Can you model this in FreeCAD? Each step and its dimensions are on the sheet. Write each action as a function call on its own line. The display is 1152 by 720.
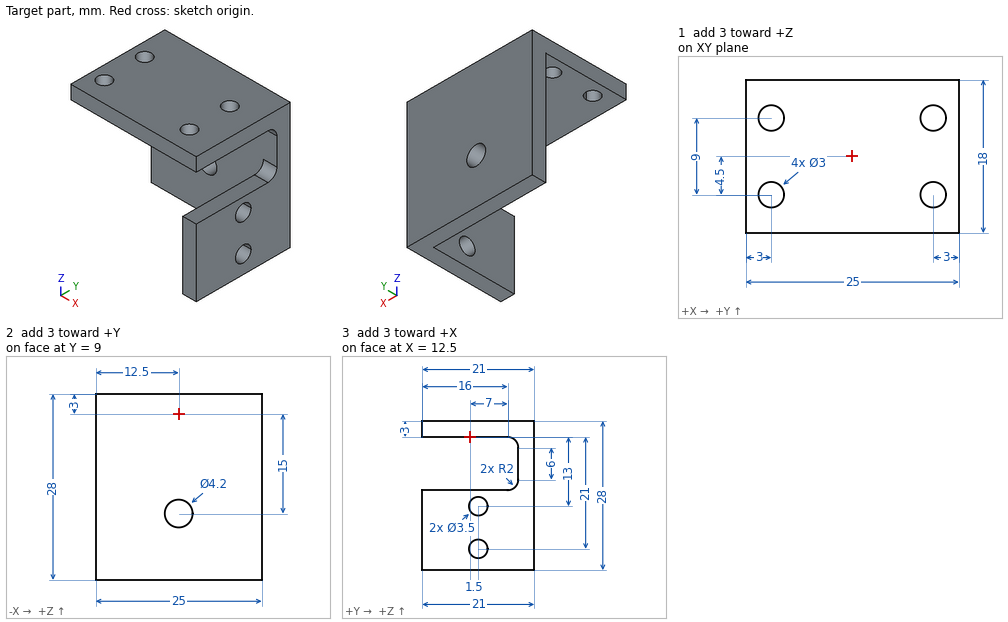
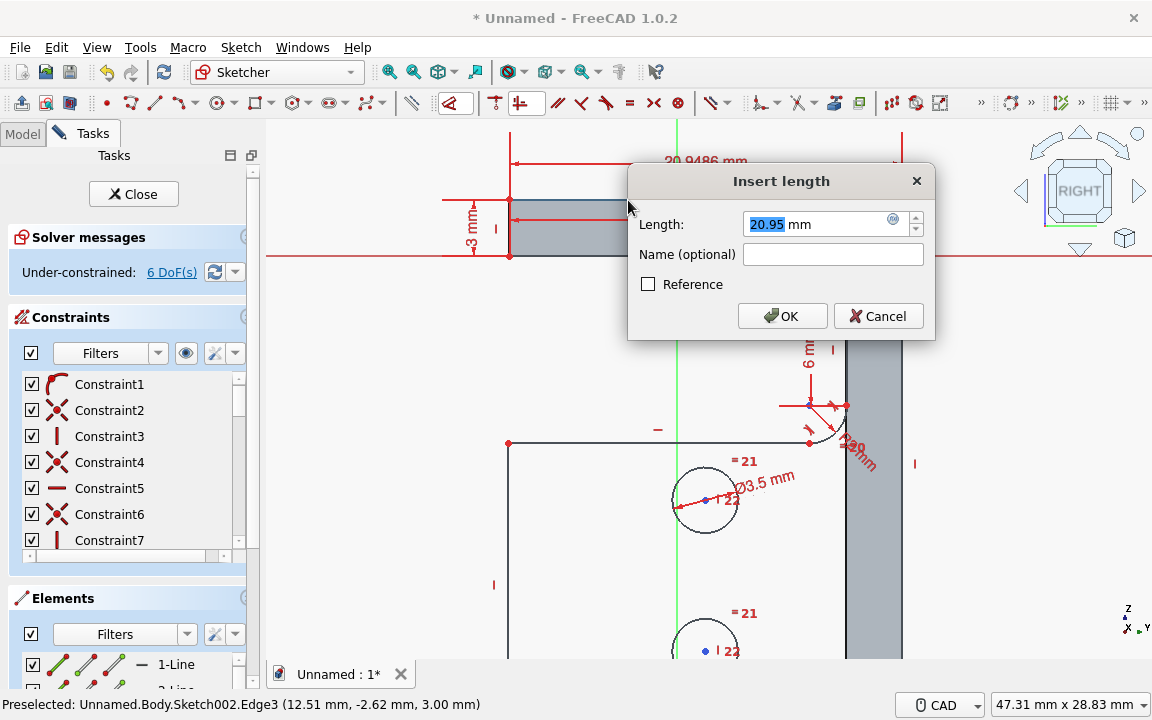
text(21)
key(Return)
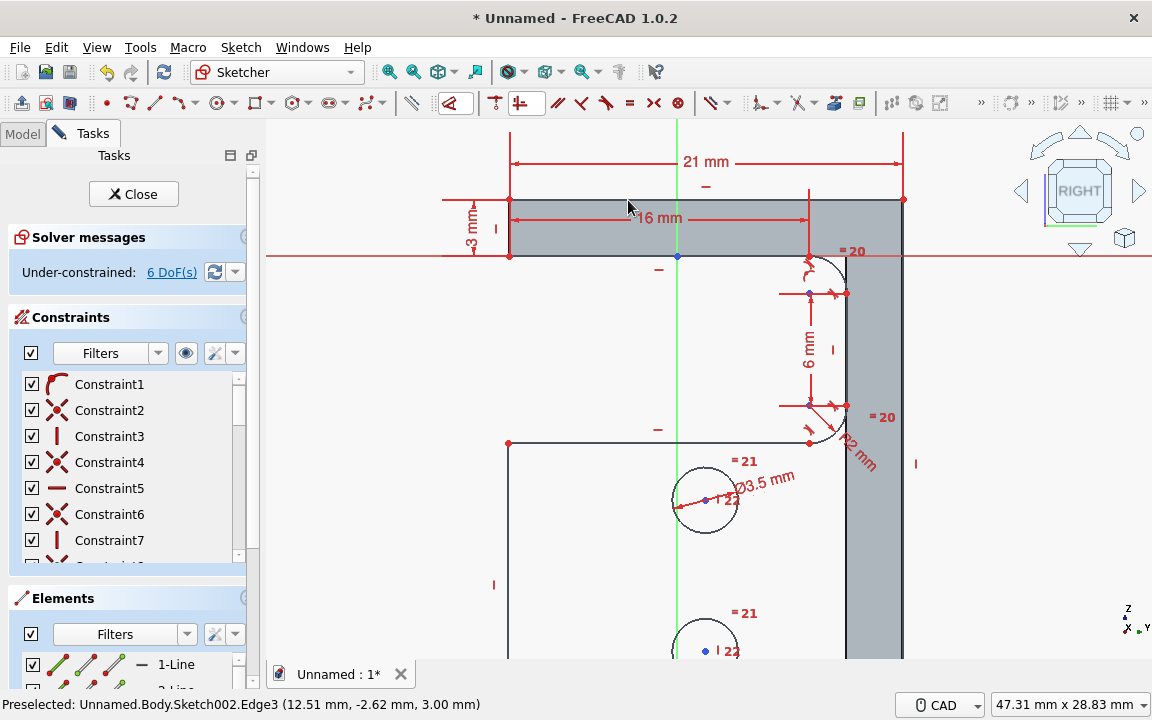
click(903, 358)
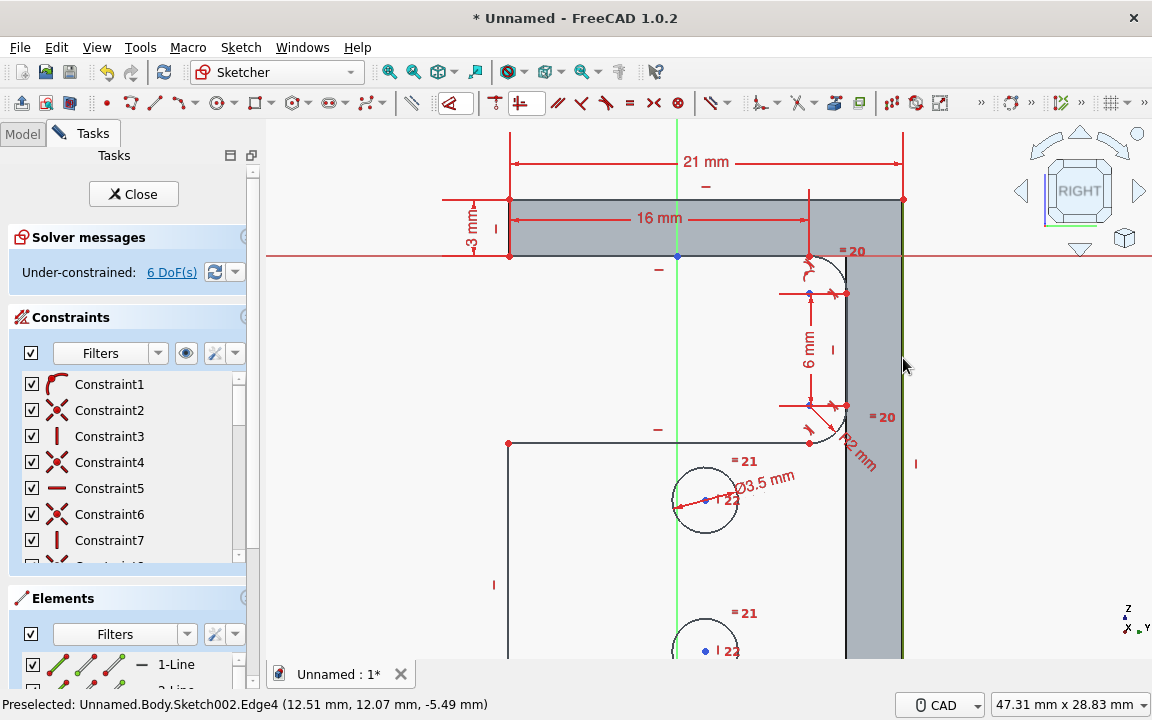
key(i)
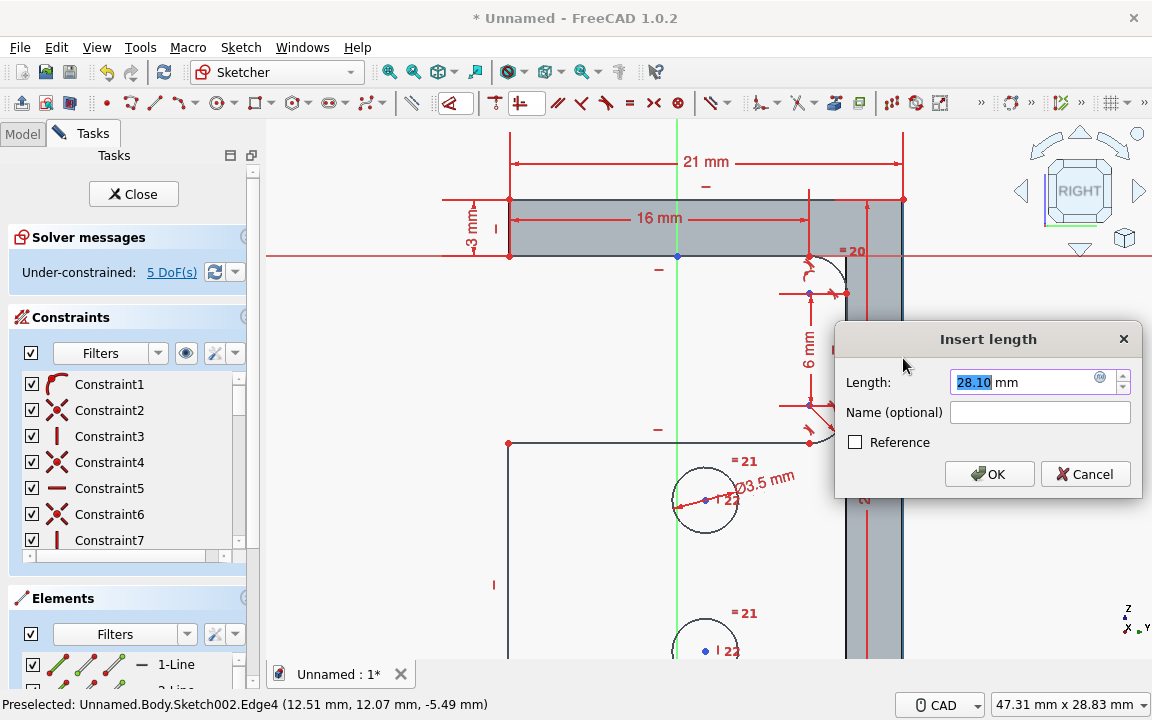
text(28)
key(Return)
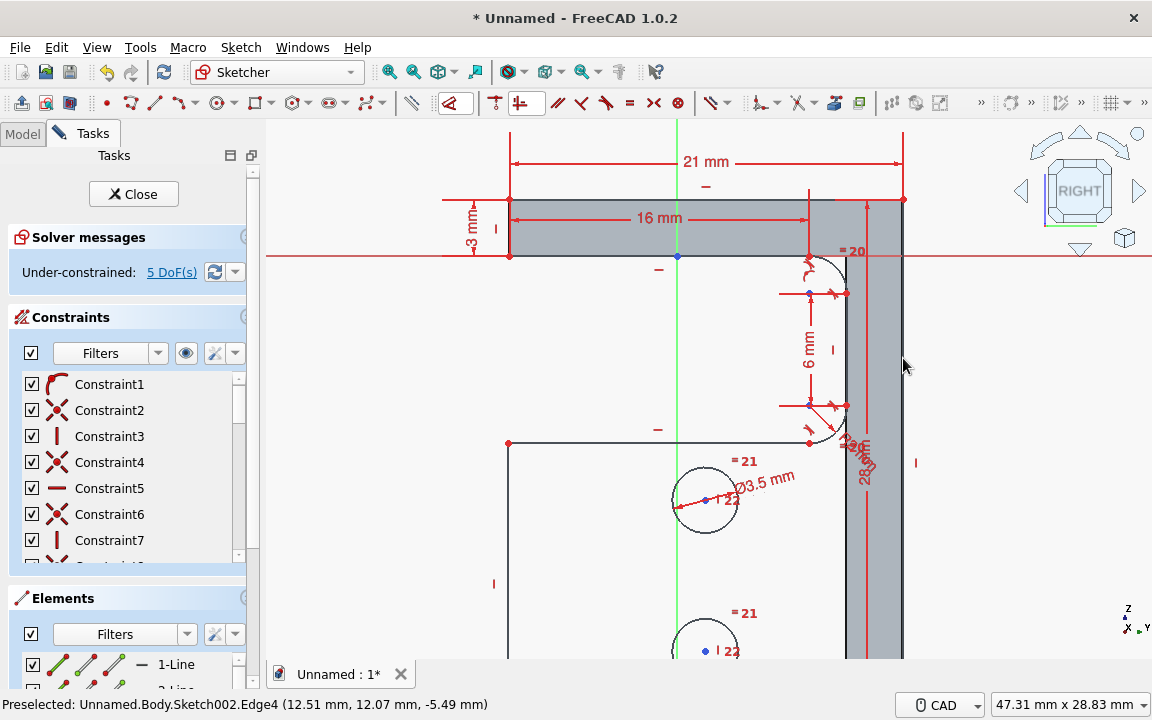
scroll(509, 240, down, 2)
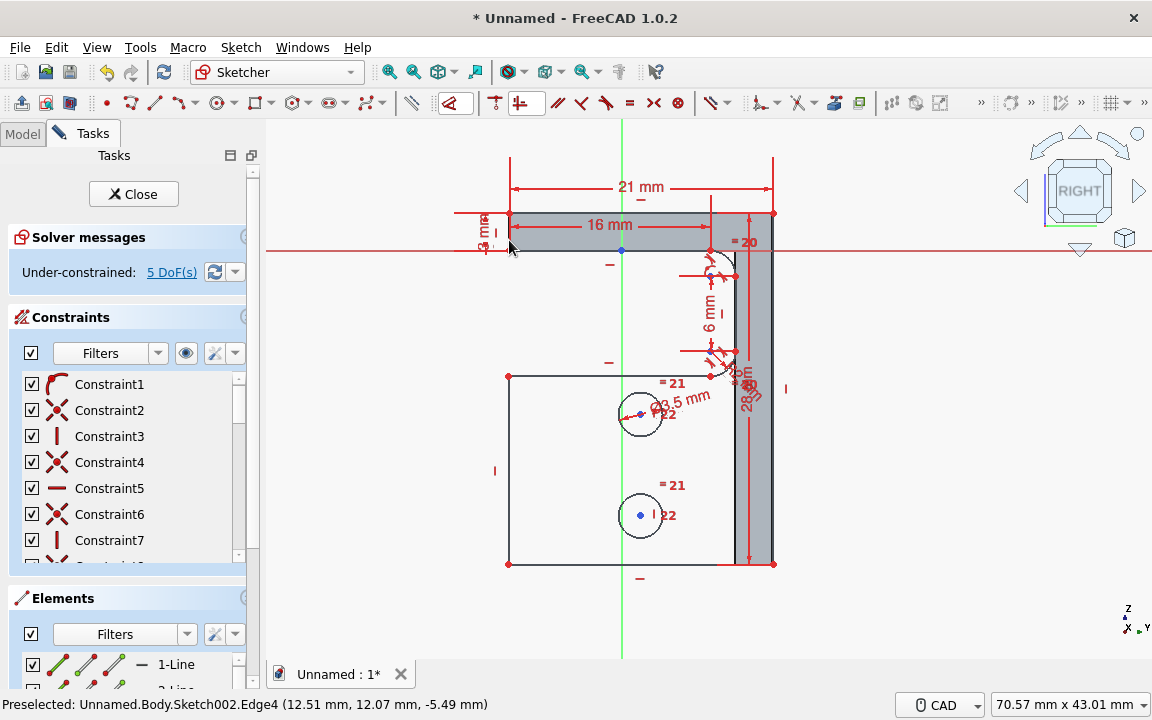
click(694, 565)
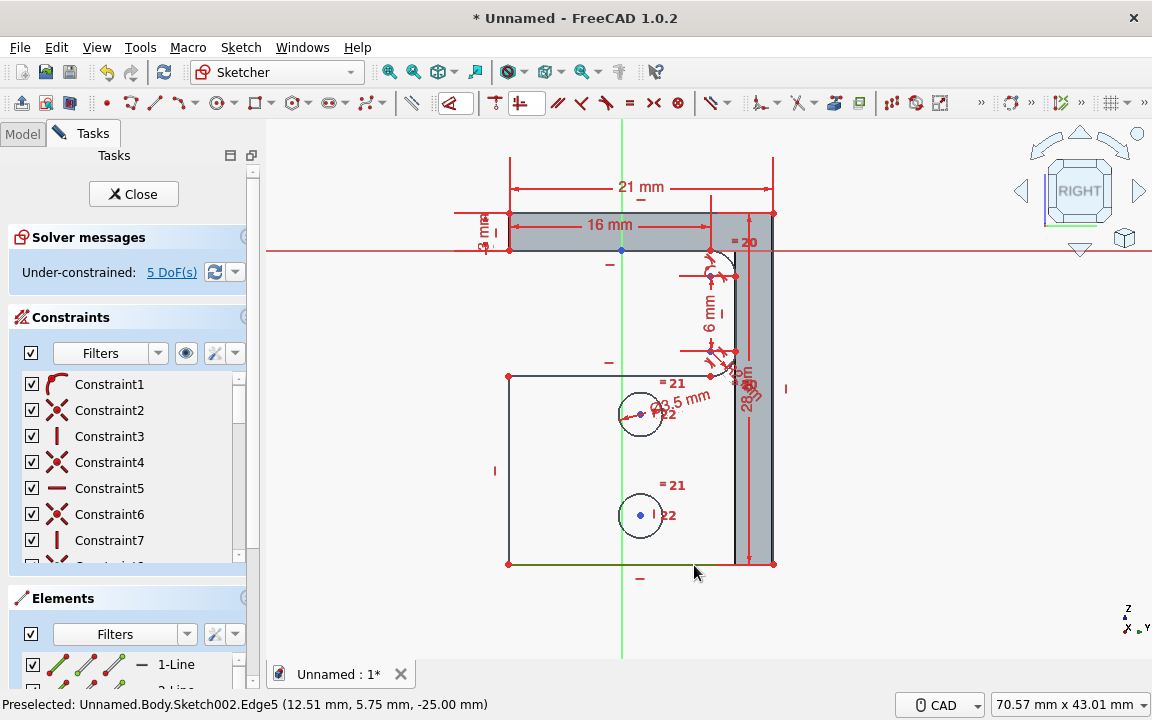
key(l)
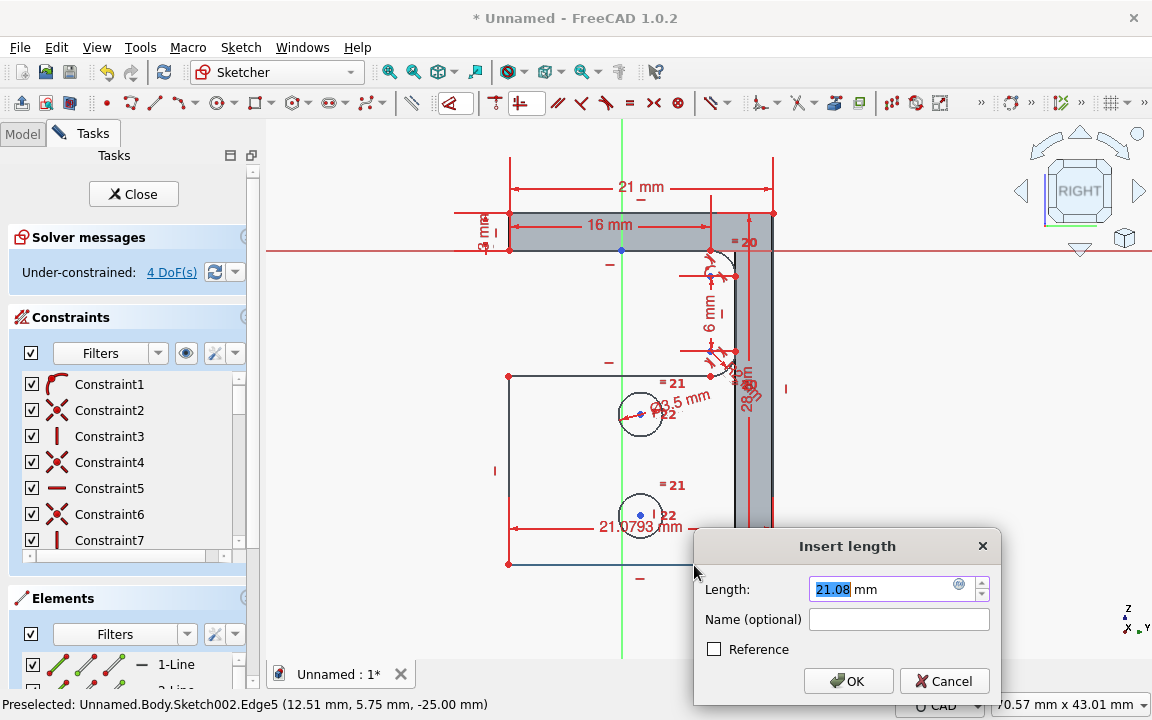
text(21)
key(Return)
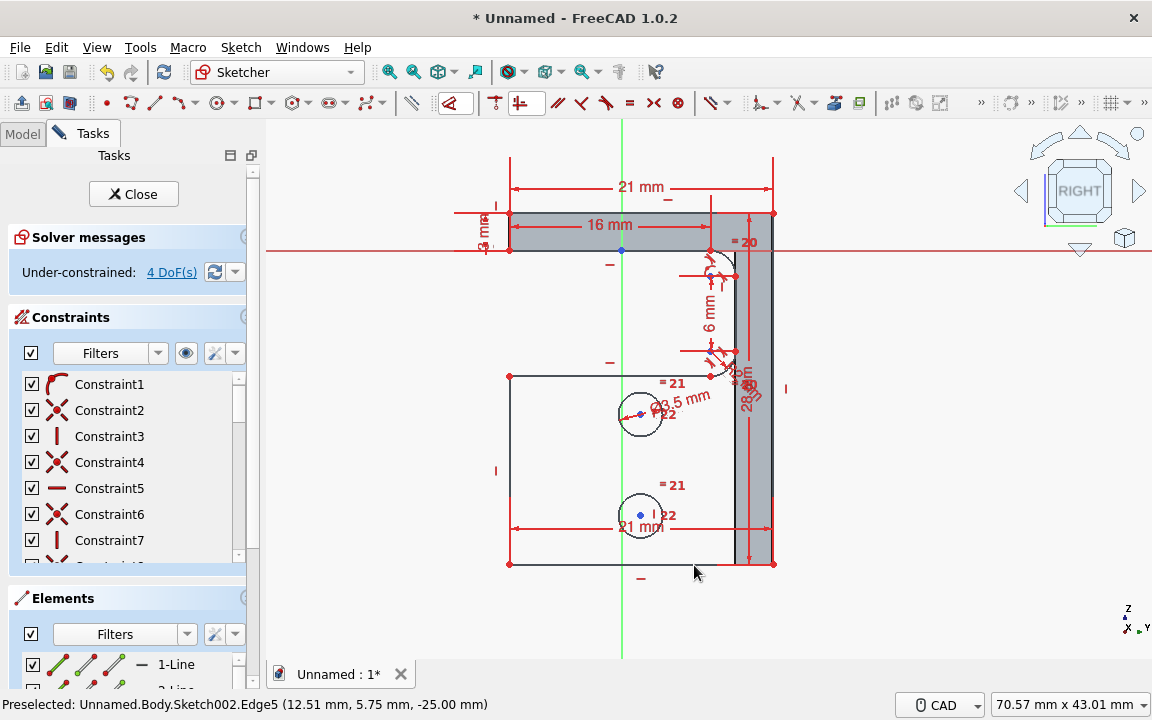
click(711, 251)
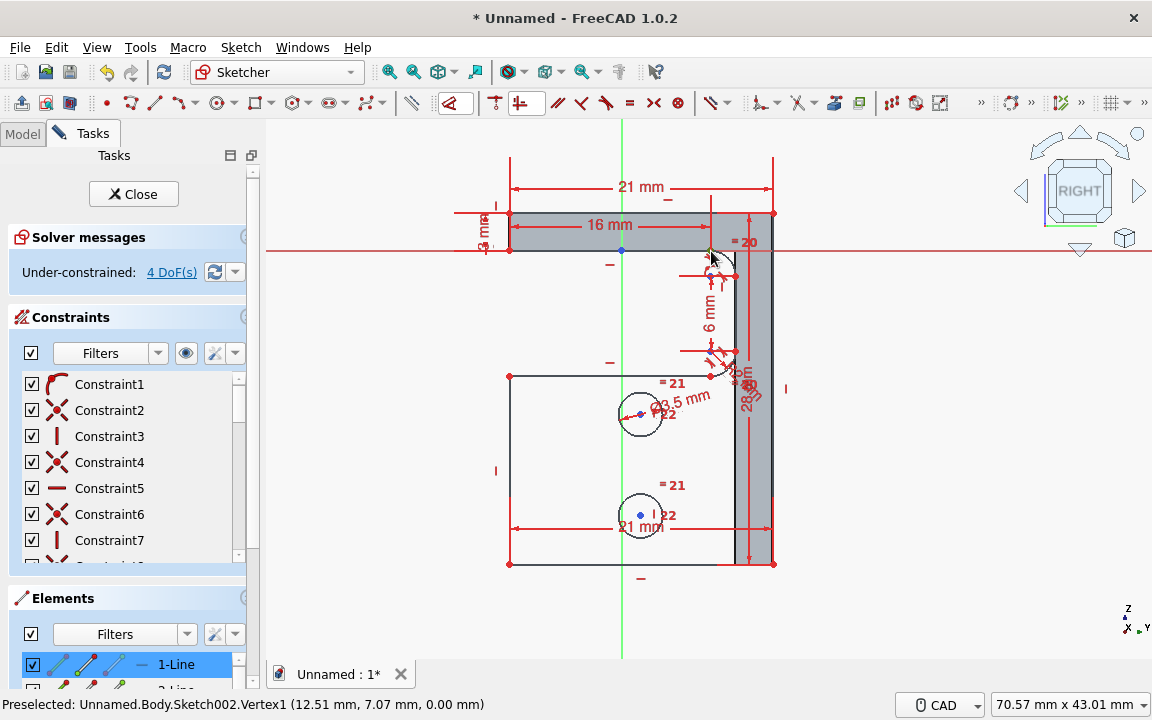
click(468, 104)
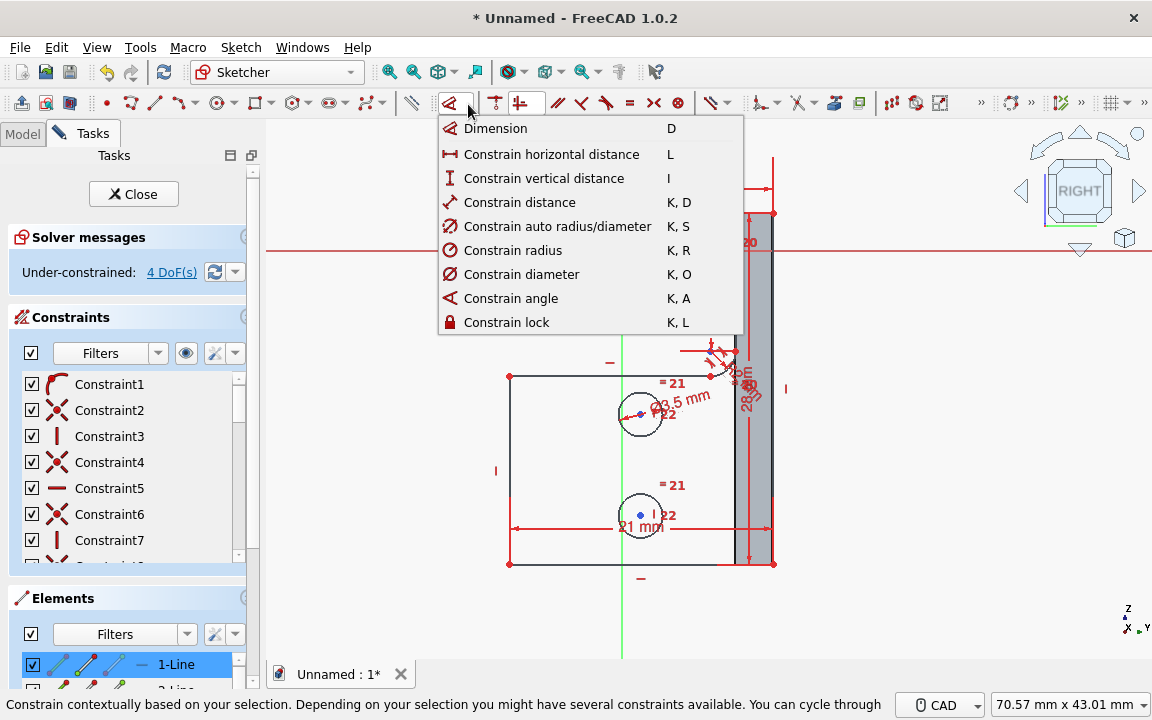
click(591, 154)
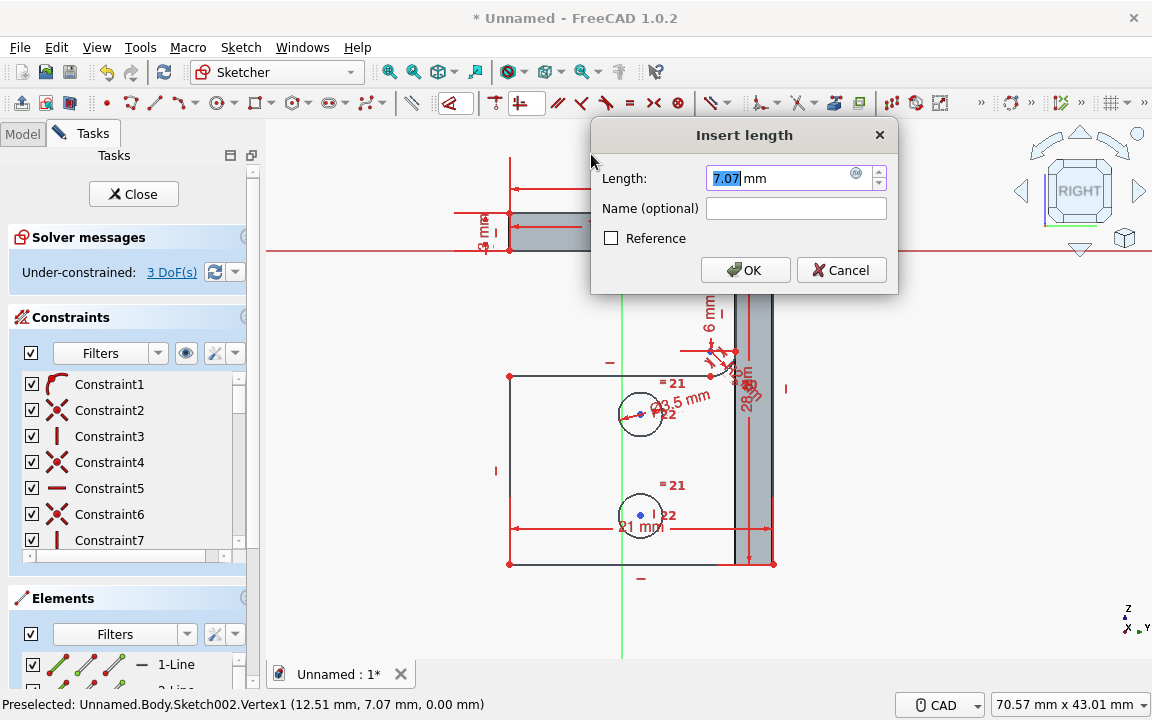
text(7)
key(Return)